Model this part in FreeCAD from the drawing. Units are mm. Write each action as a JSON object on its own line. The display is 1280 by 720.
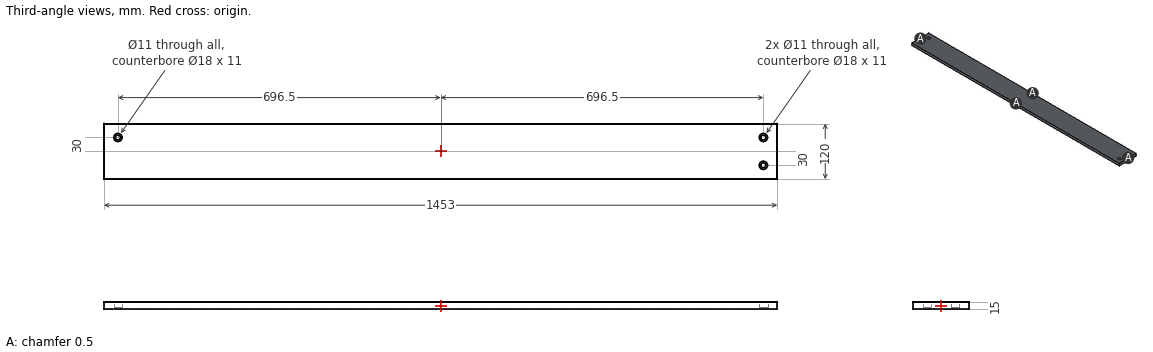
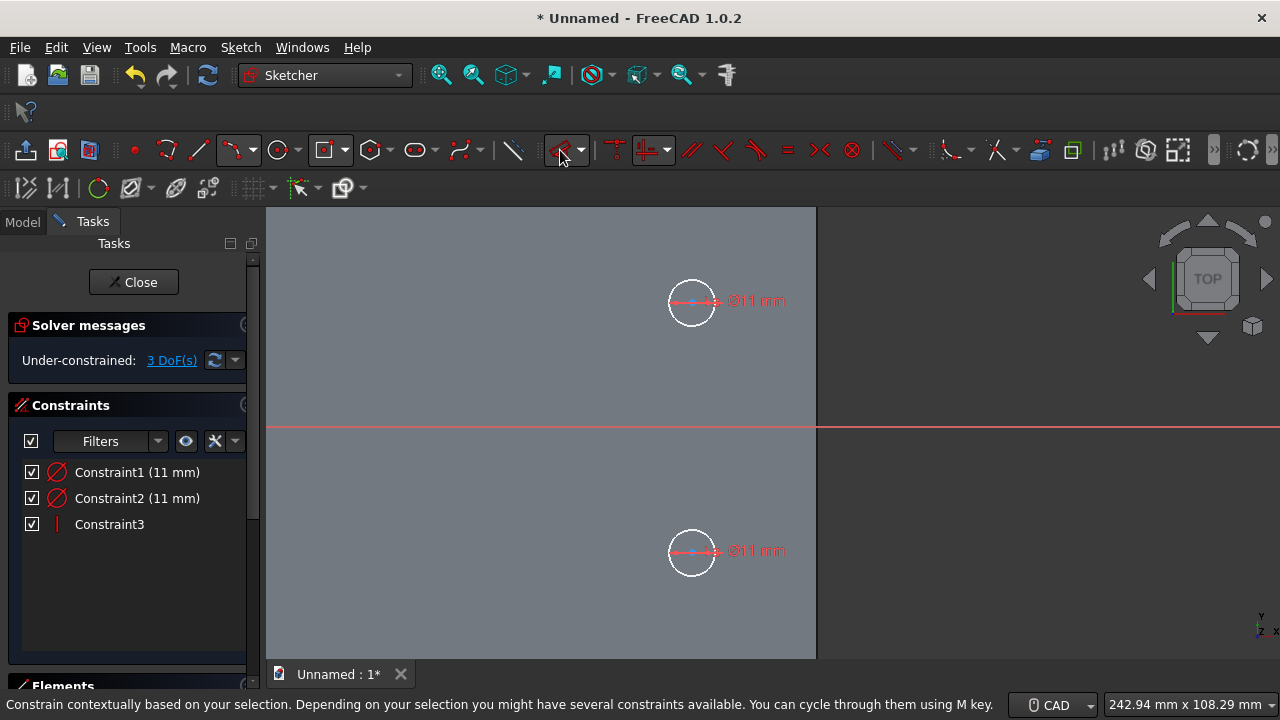
{"action": "left_click", "coordinate": [692, 303]}
{"action": "left_click", "coordinate": [726, 365]}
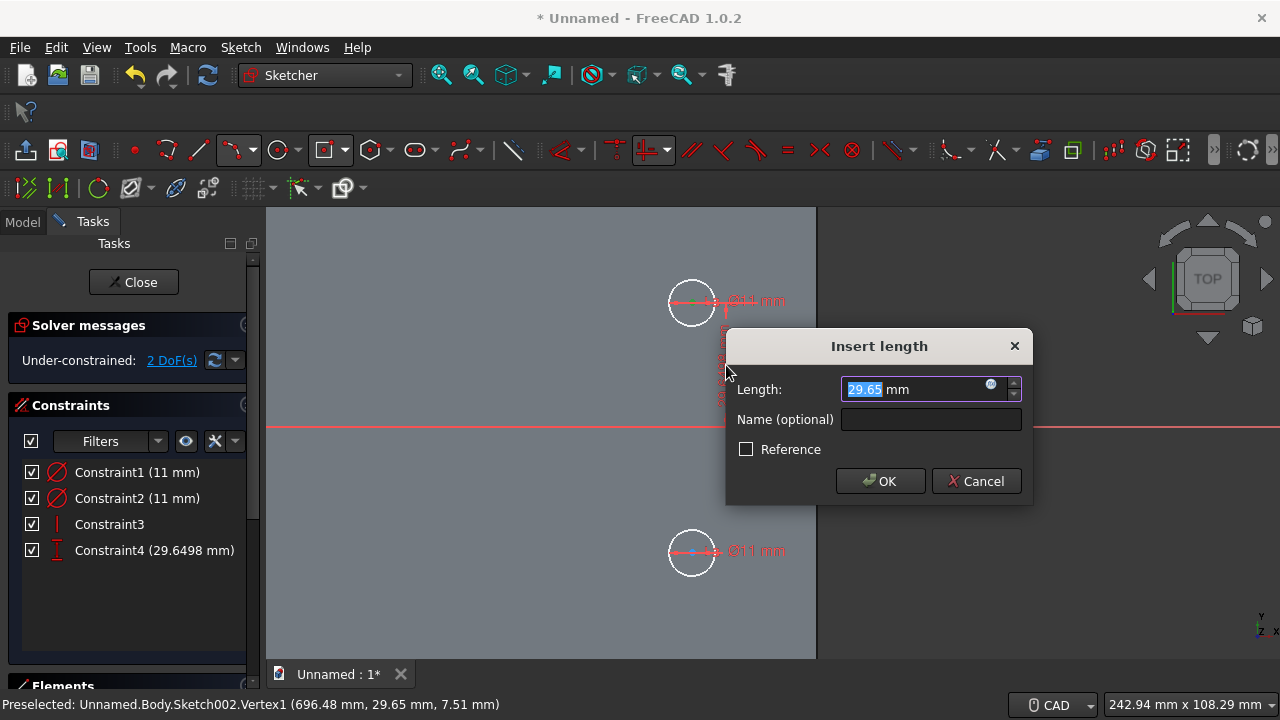
{"action": "type", "text": "30"}
{"action": "key", "text": "Return"}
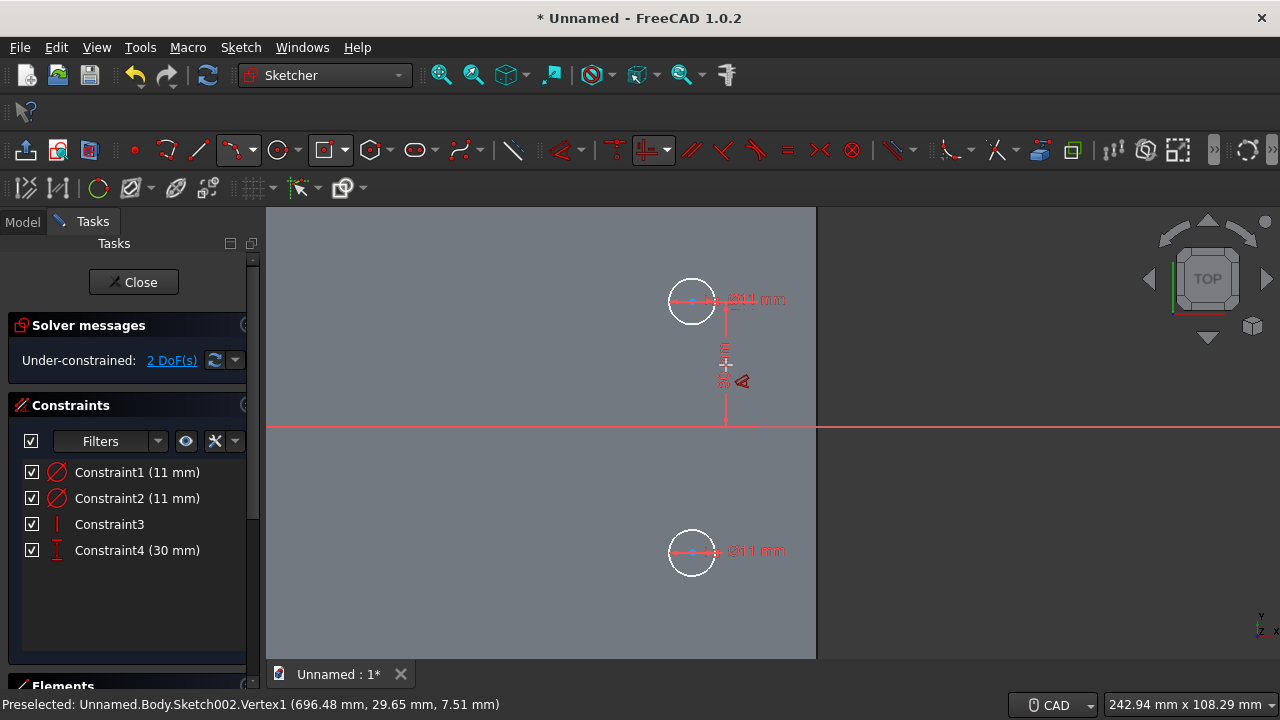
{"action": "left_click", "coordinate": [692, 553]}
{"action": "left_click", "coordinate": [726, 490]}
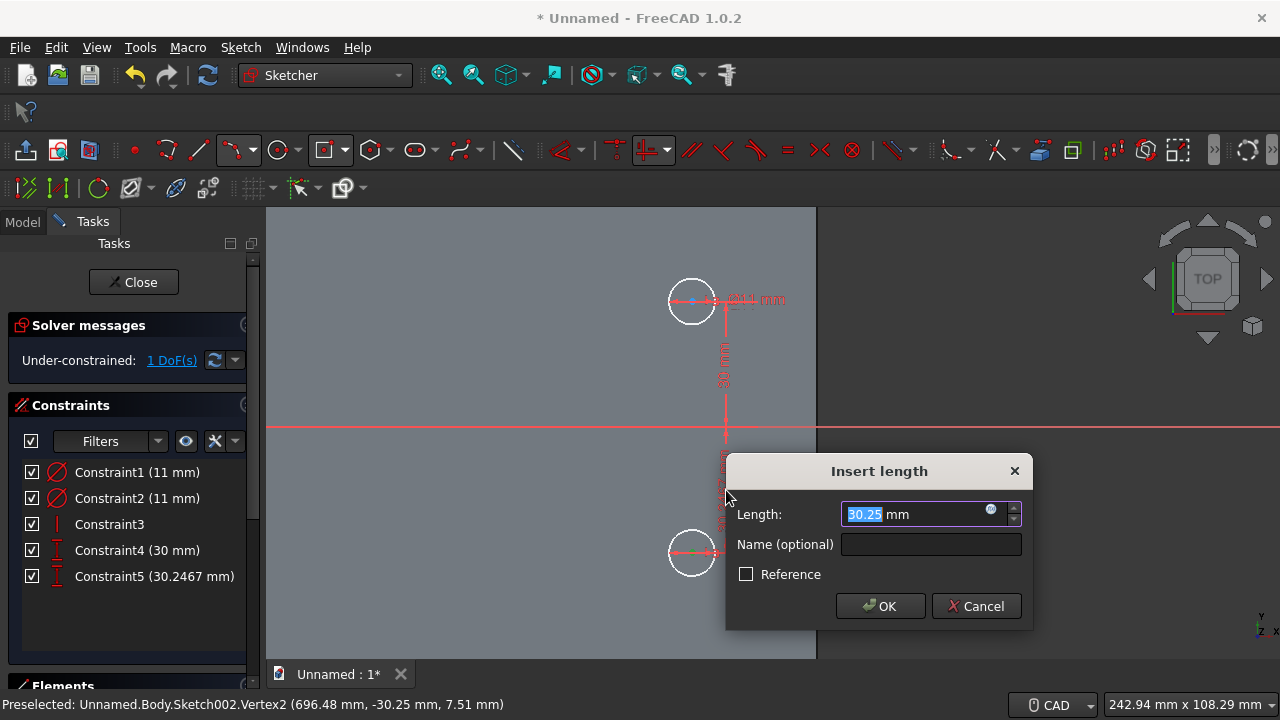
{"action": "type", "text": "30"}
{"action": "key", "text": "Return"}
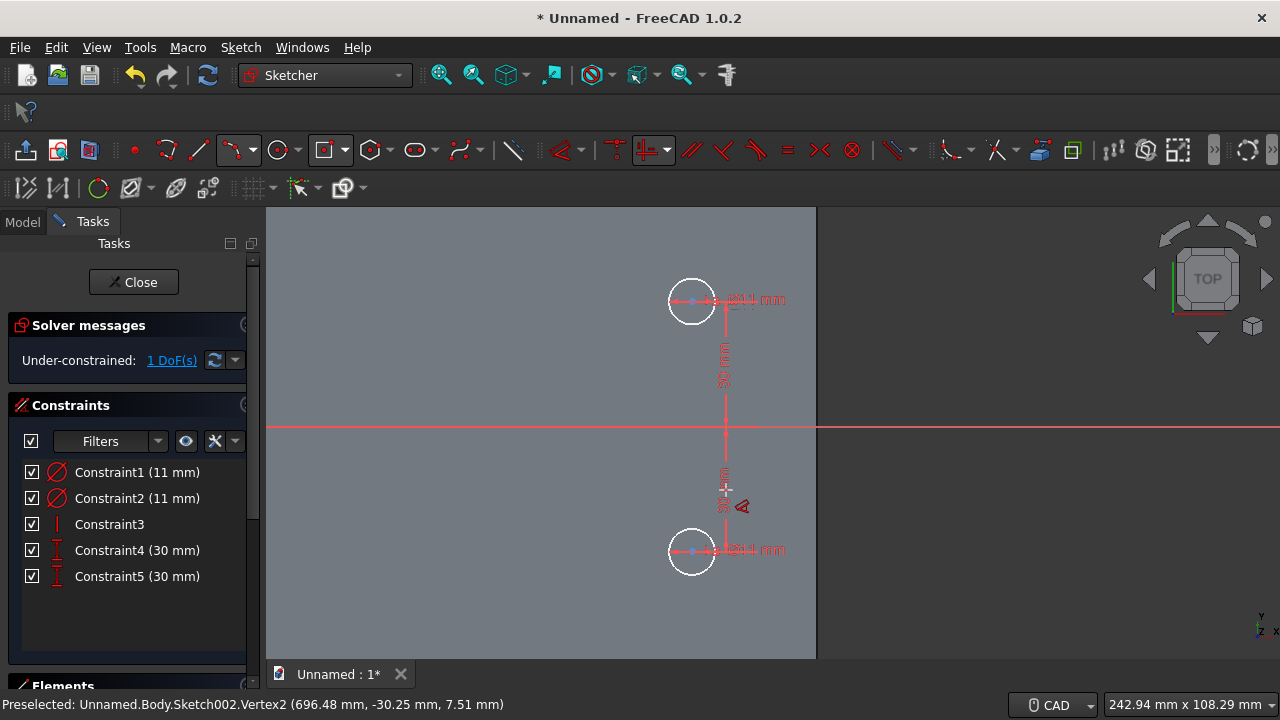
{"action": "left_click", "coordinate": [692, 302]}
{"action": "left_click", "coordinate": [493, 268]}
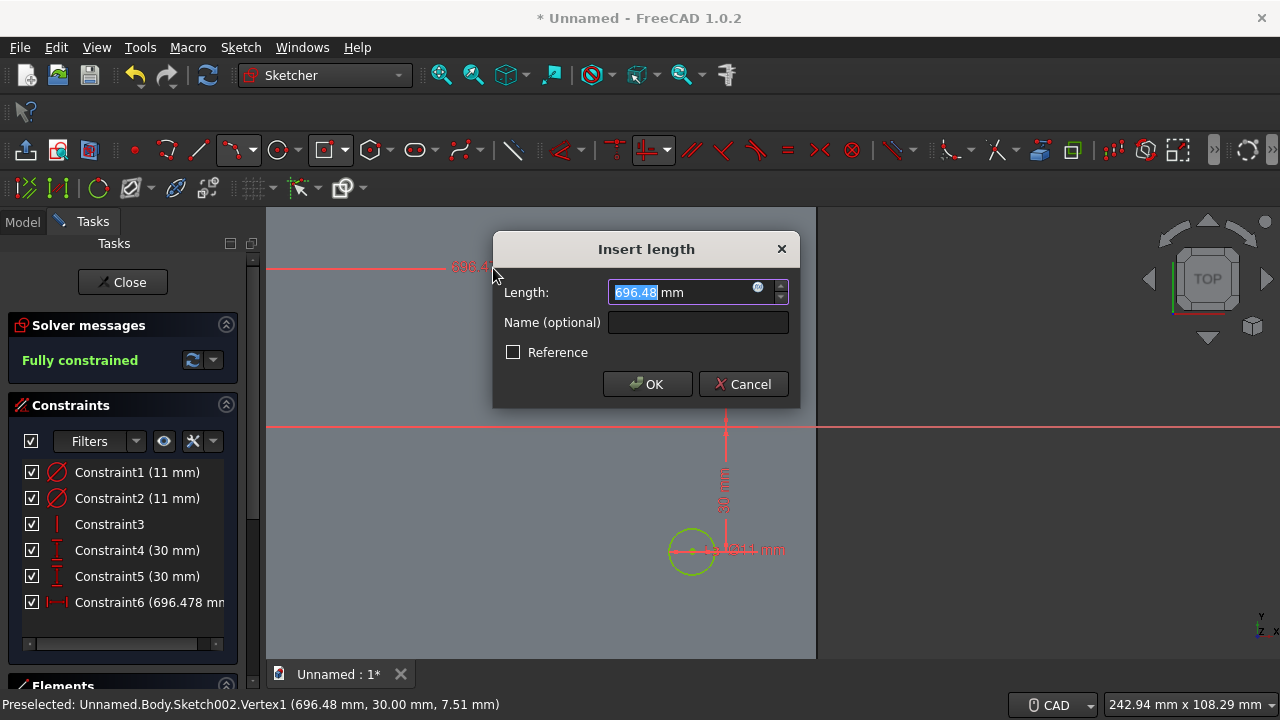
{"action": "type", "text": "696.5"}
{"action": "key", "text": "Return"}
{"action": "key", "text": "Escape"}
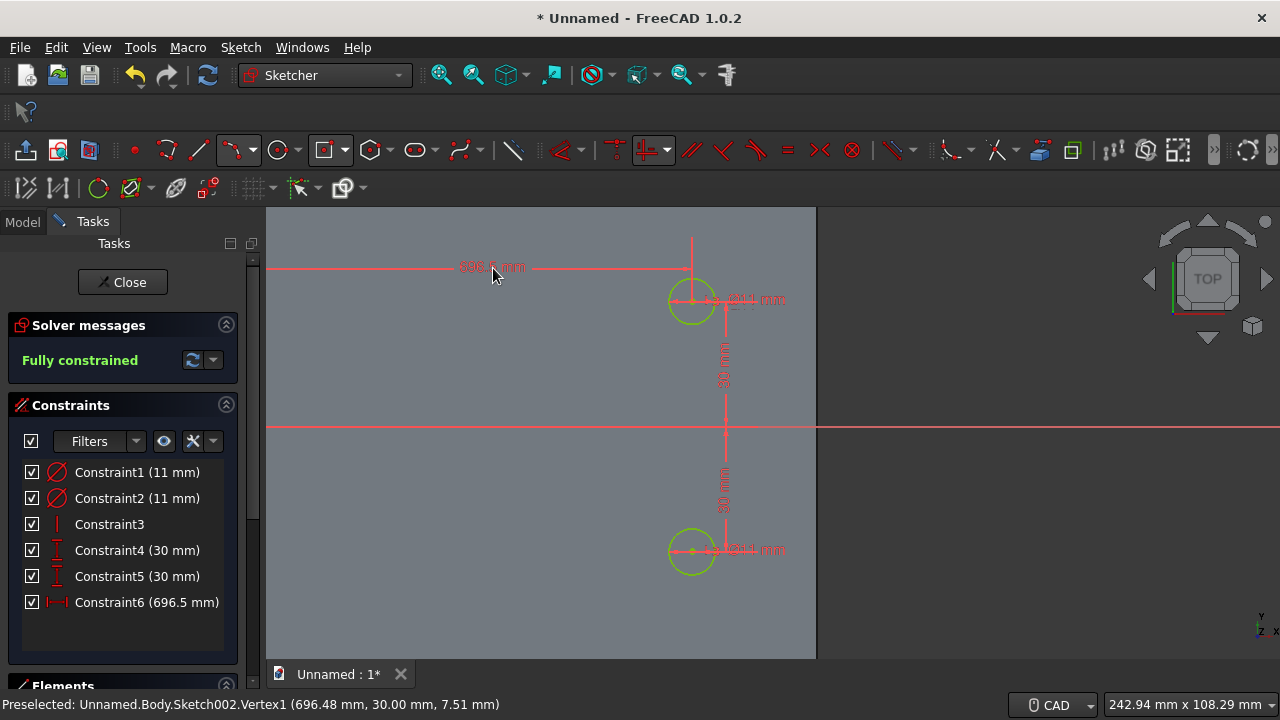
{"action": "left_click", "coordinate": [123, 282]}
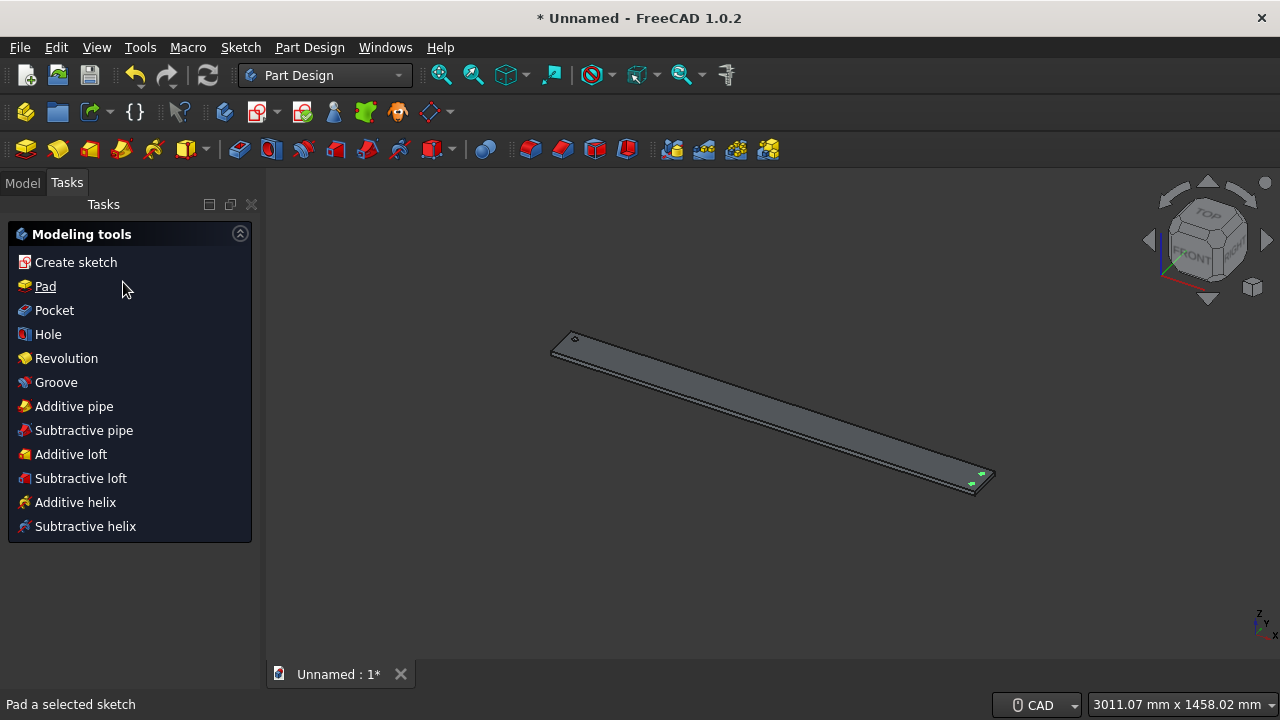
{"action": "left_click", "coordinate": [272, 150]}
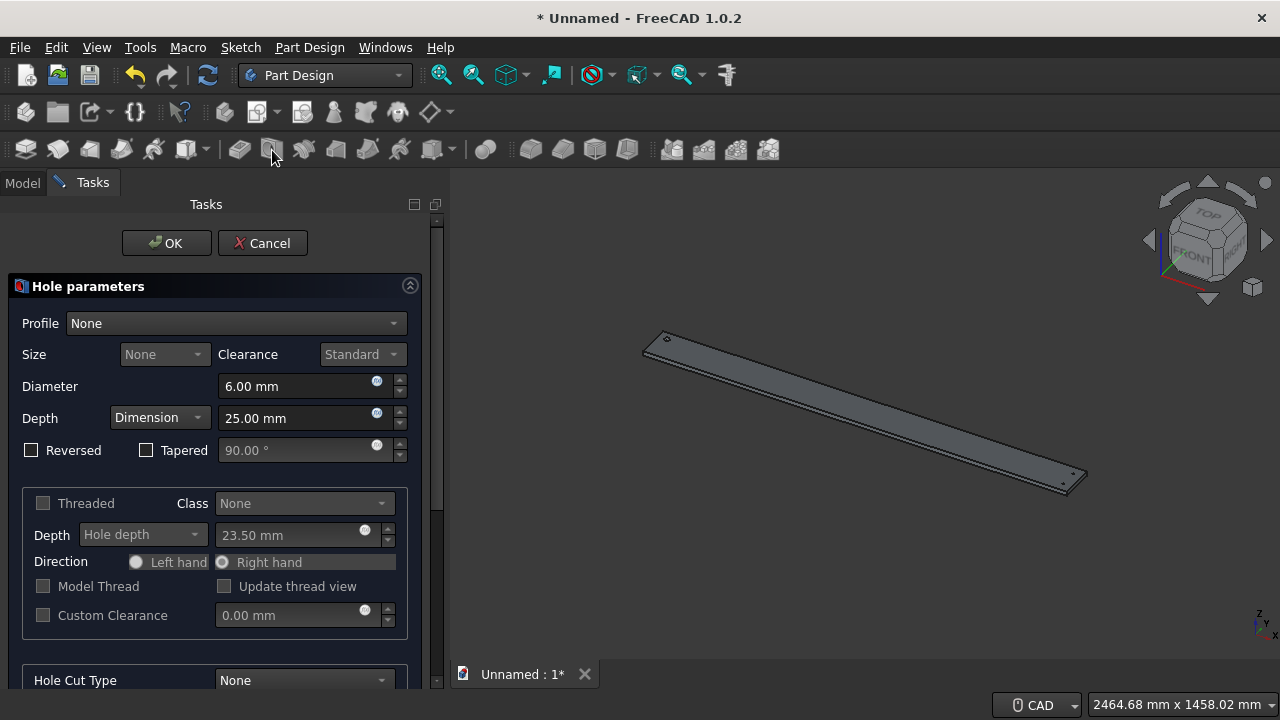
{"action": "triple_click", "coordinate": [305, 386]}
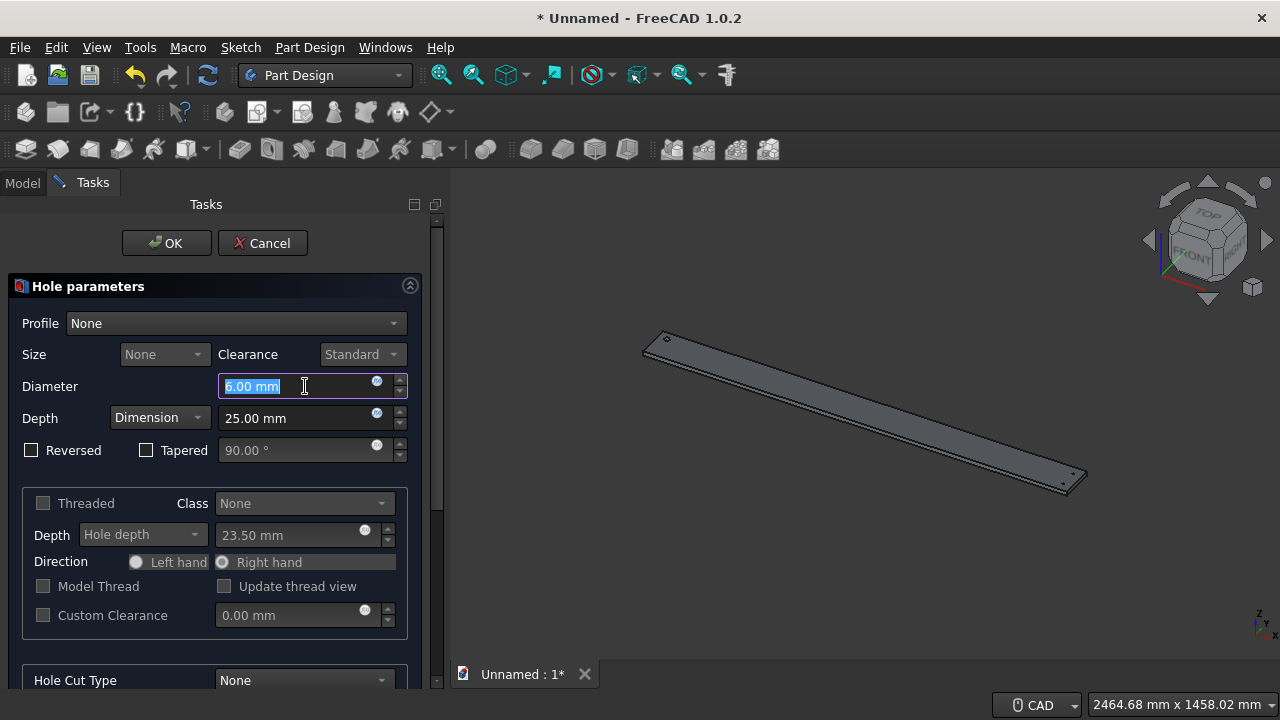
{"action": "type", "text": "11"}
{"action": "key", "text": "Tab"}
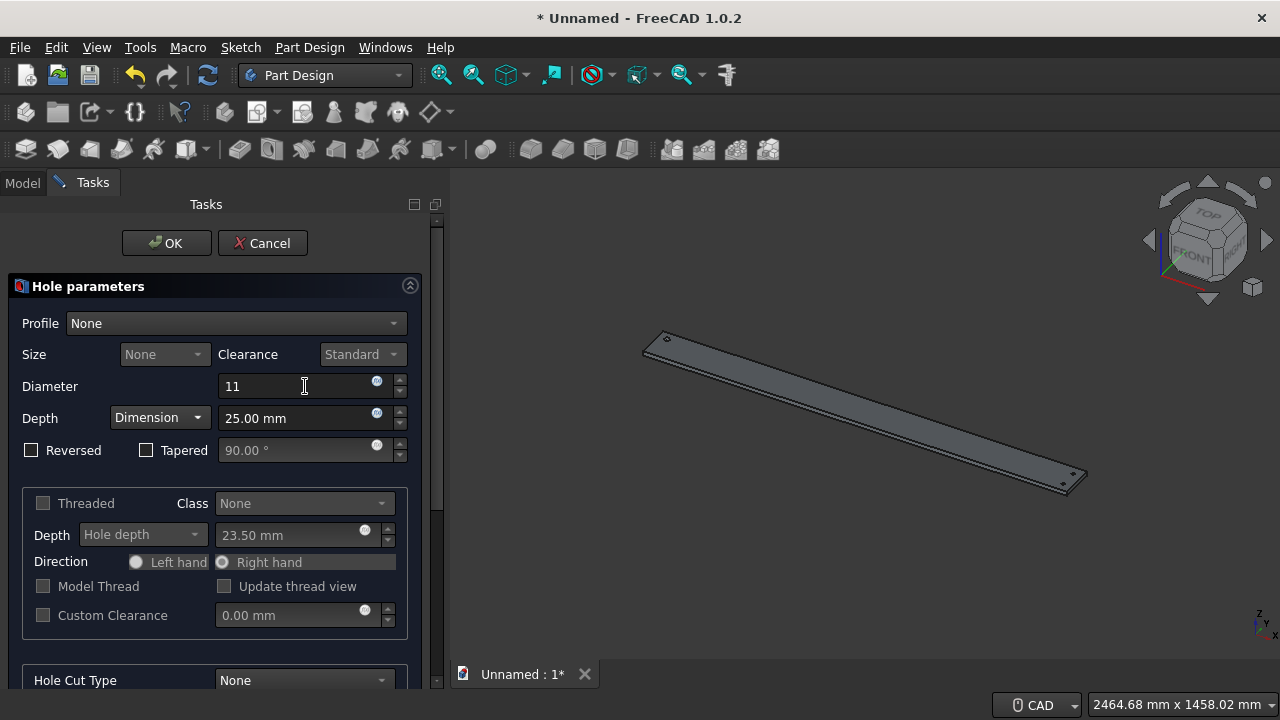
{"action": "left_click", "coordinate": [161, 418]}